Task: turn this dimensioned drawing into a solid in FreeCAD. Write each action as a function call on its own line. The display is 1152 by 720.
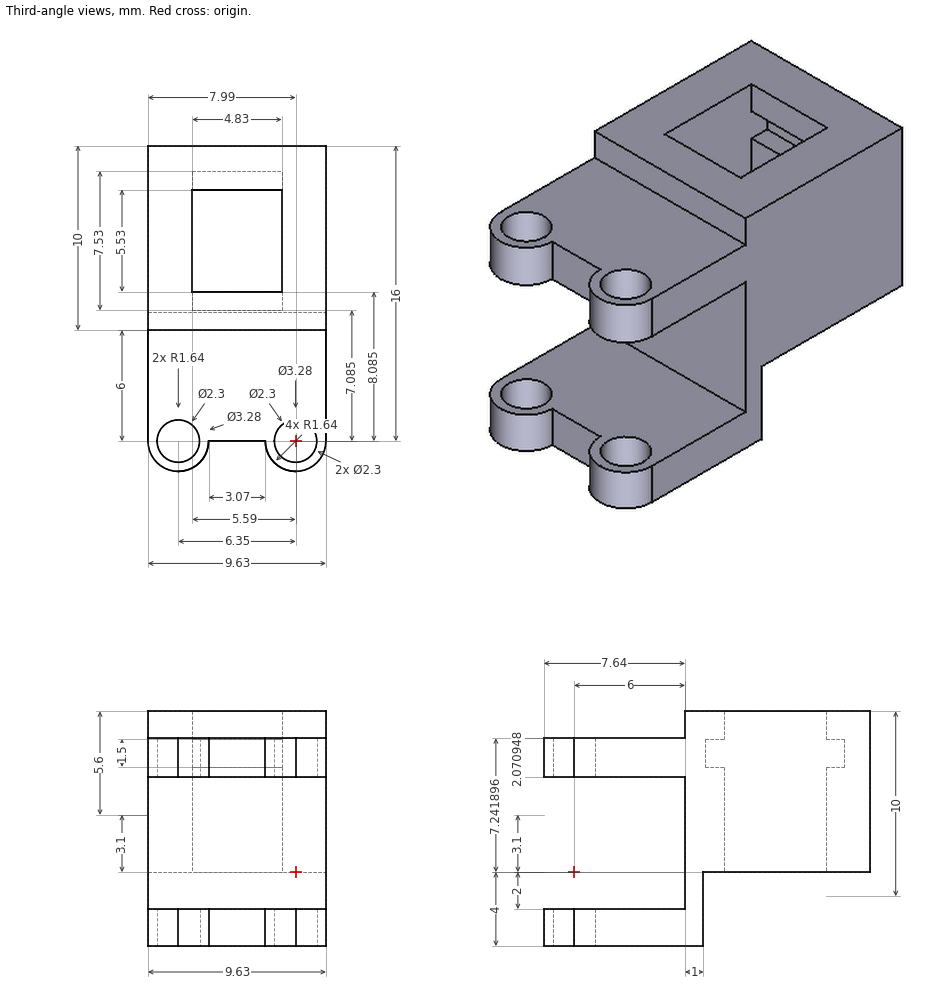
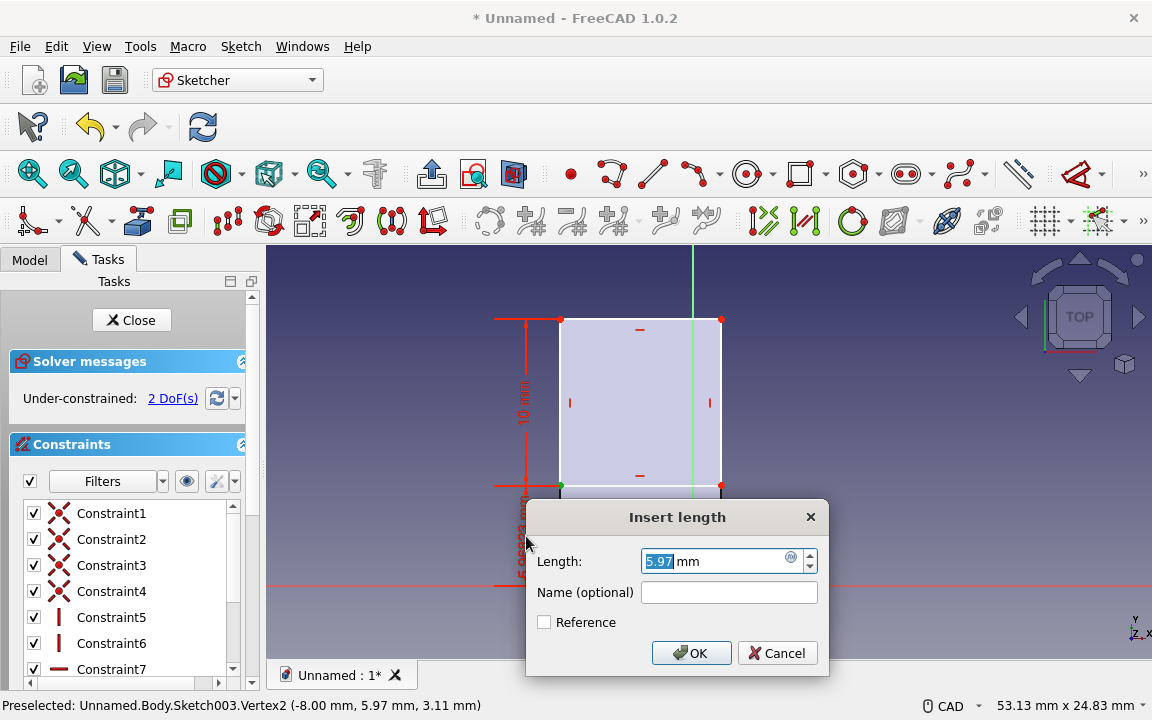
text(6)
key(Return)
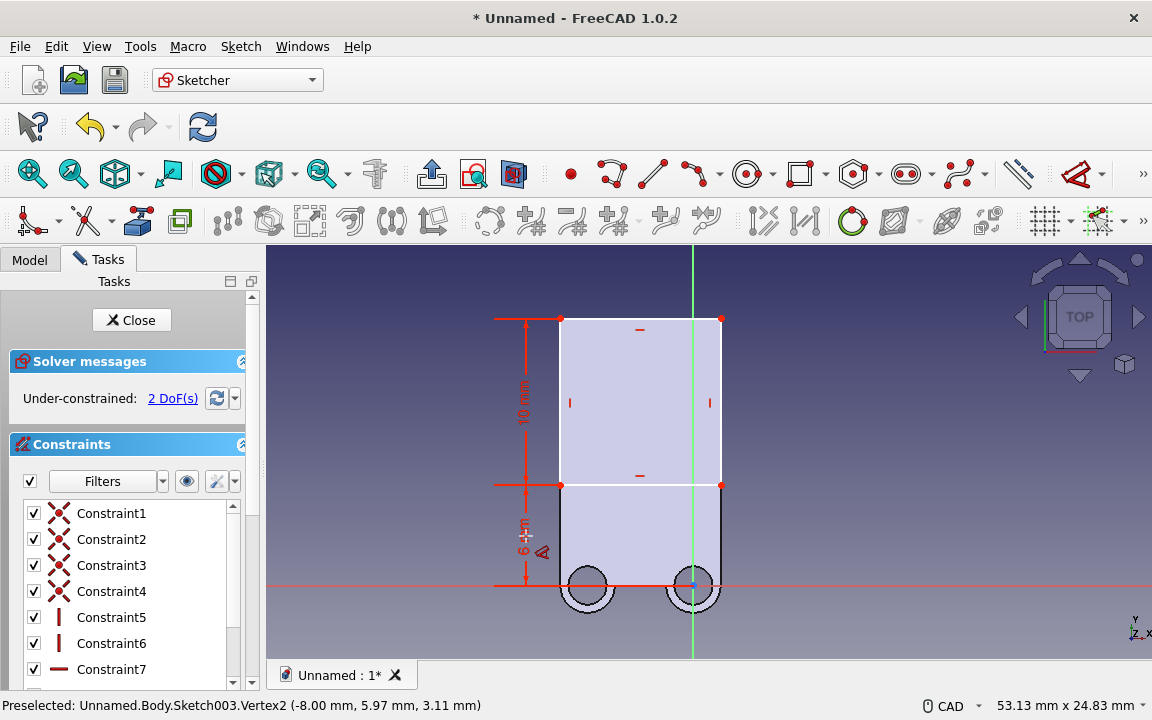
click(608, 485)
click(640, 519)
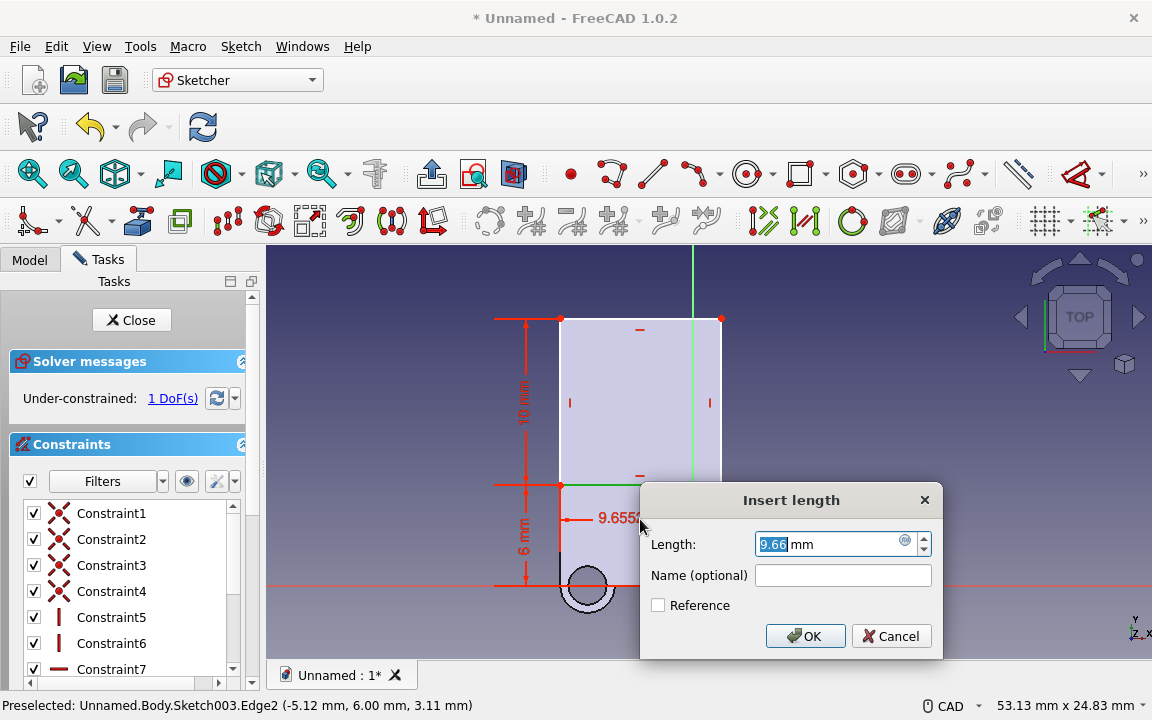
text(9.63)
key(Return)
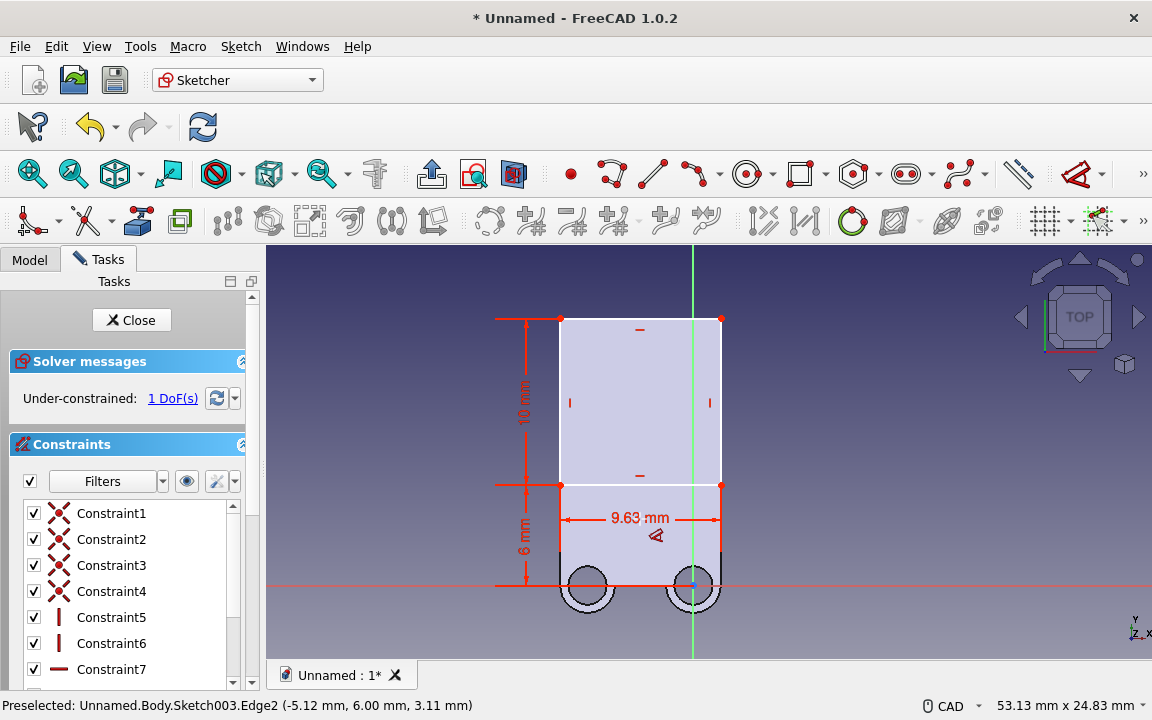
click(560, 319)
click(627, 620)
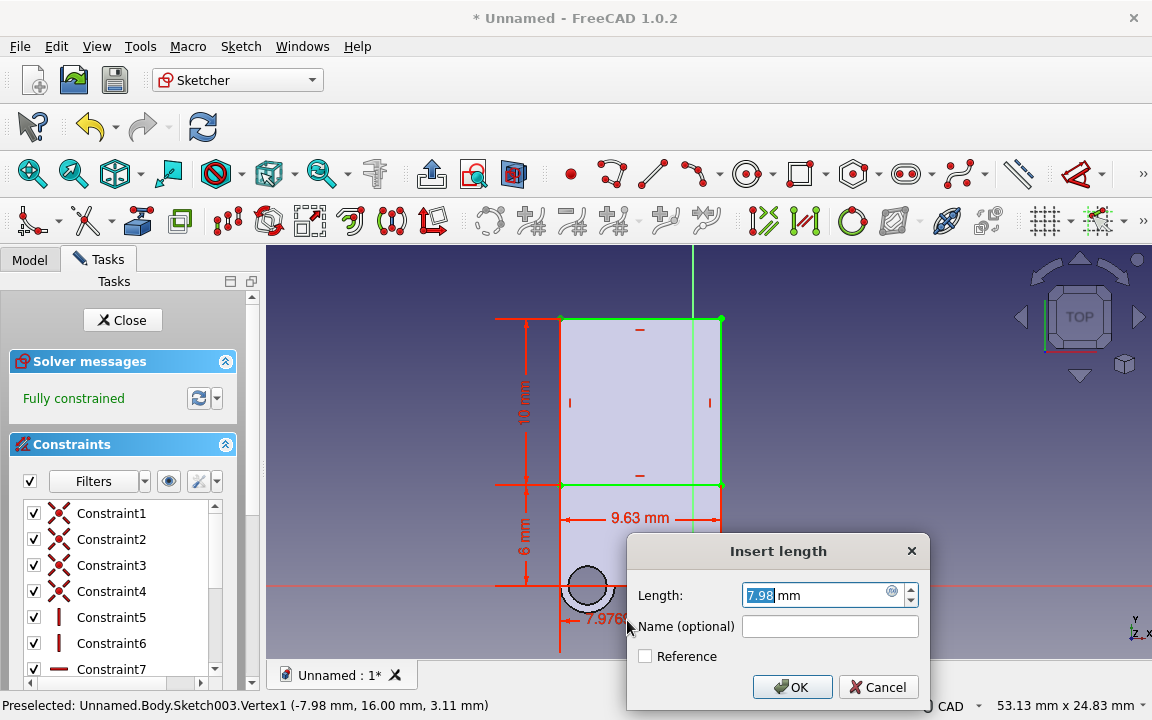
text(7.99)
key(Return)
key(Escape)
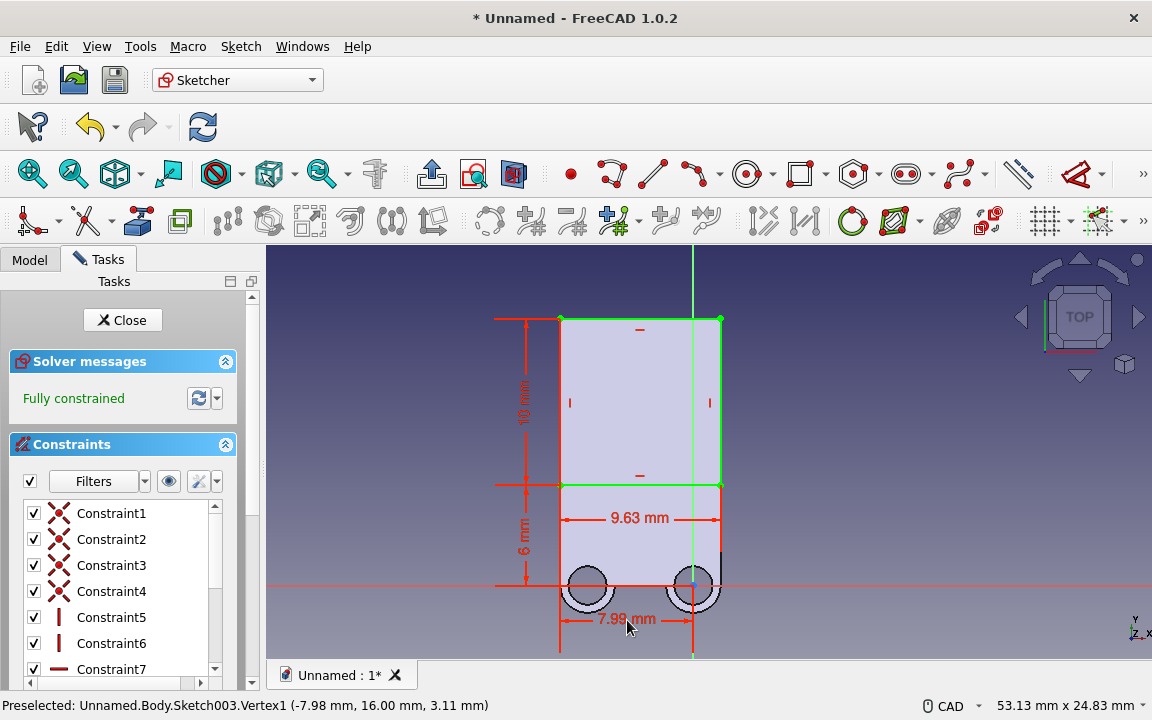
click(123, 320)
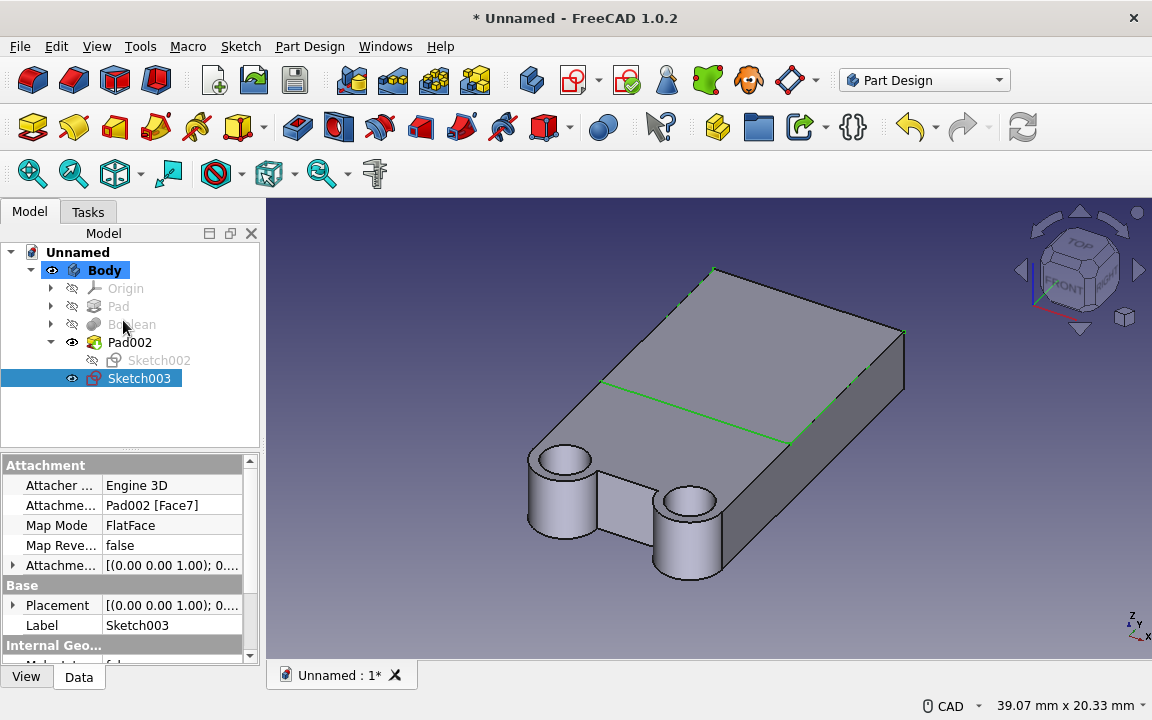
click(33, 128)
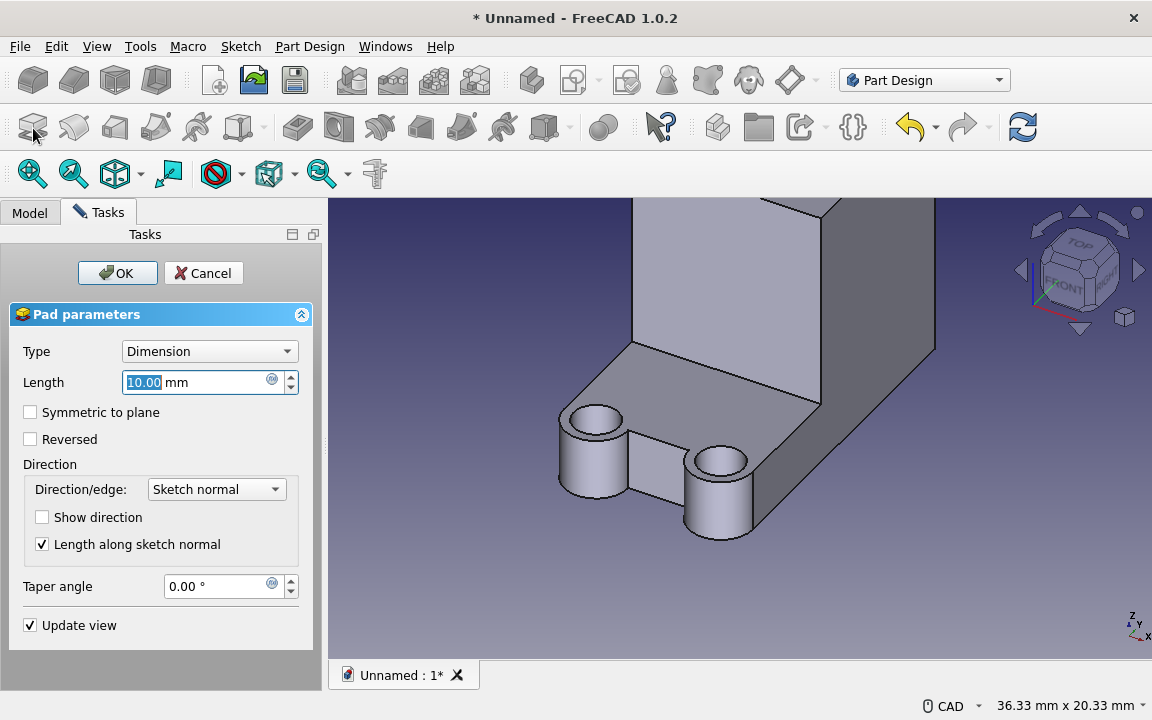
text(5.6)
key(Tab)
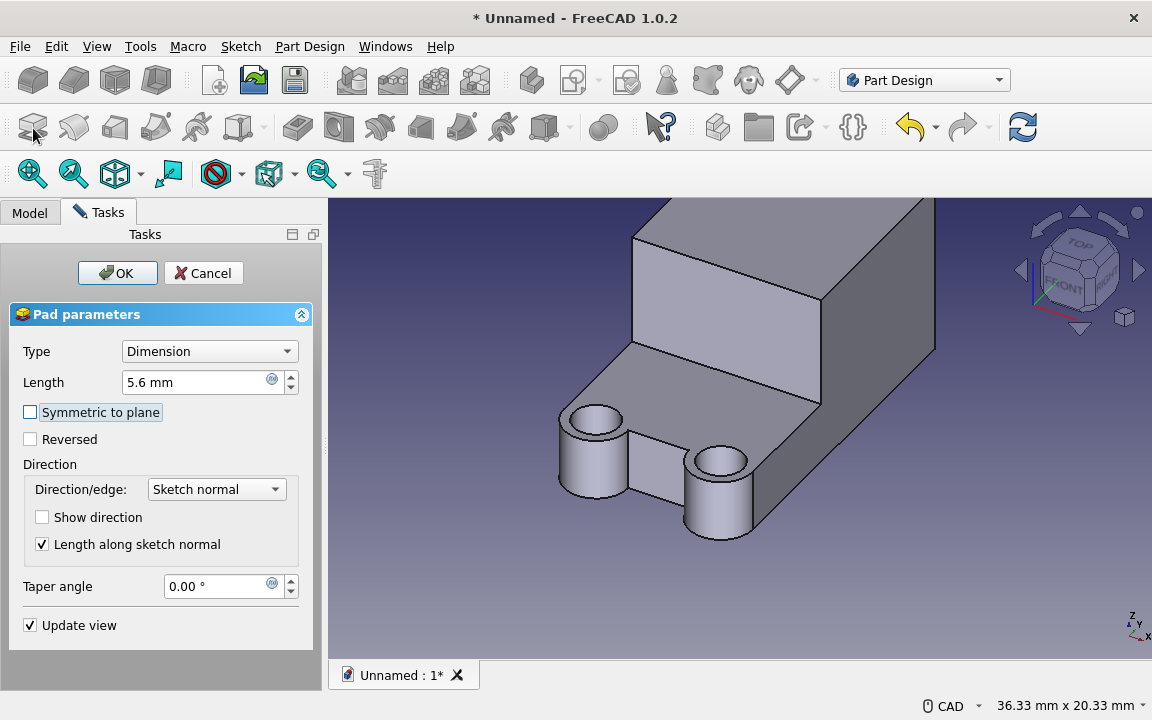
click(118, 273)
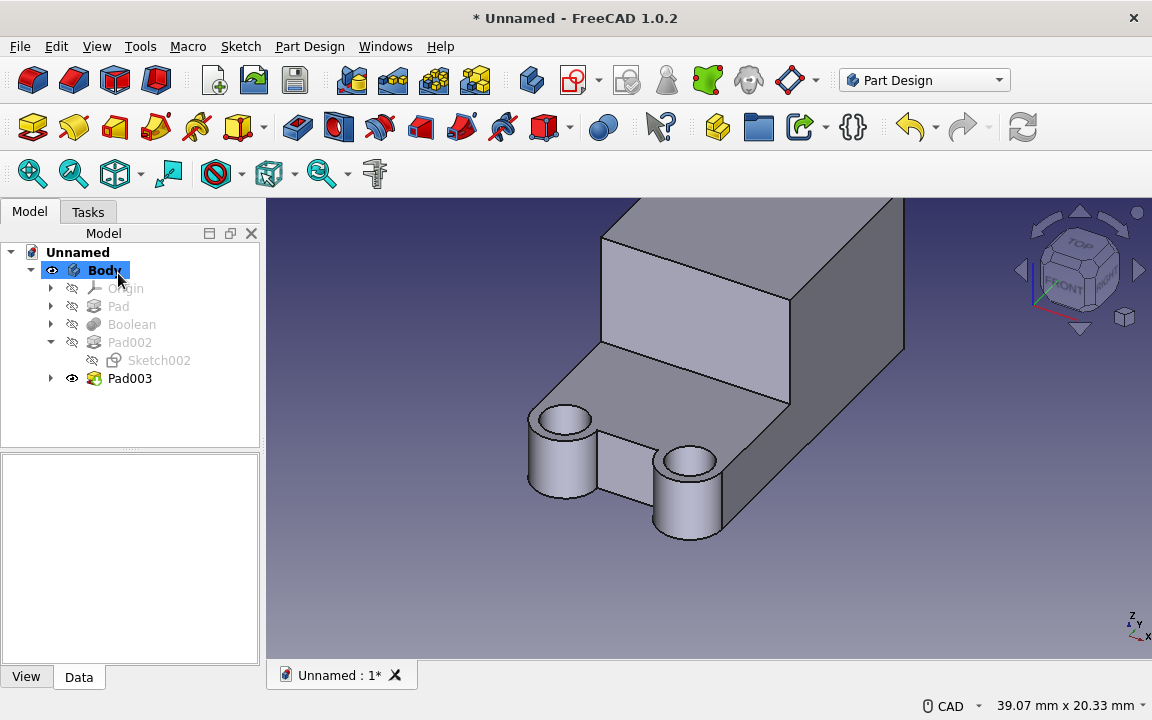
key(v)
key(f)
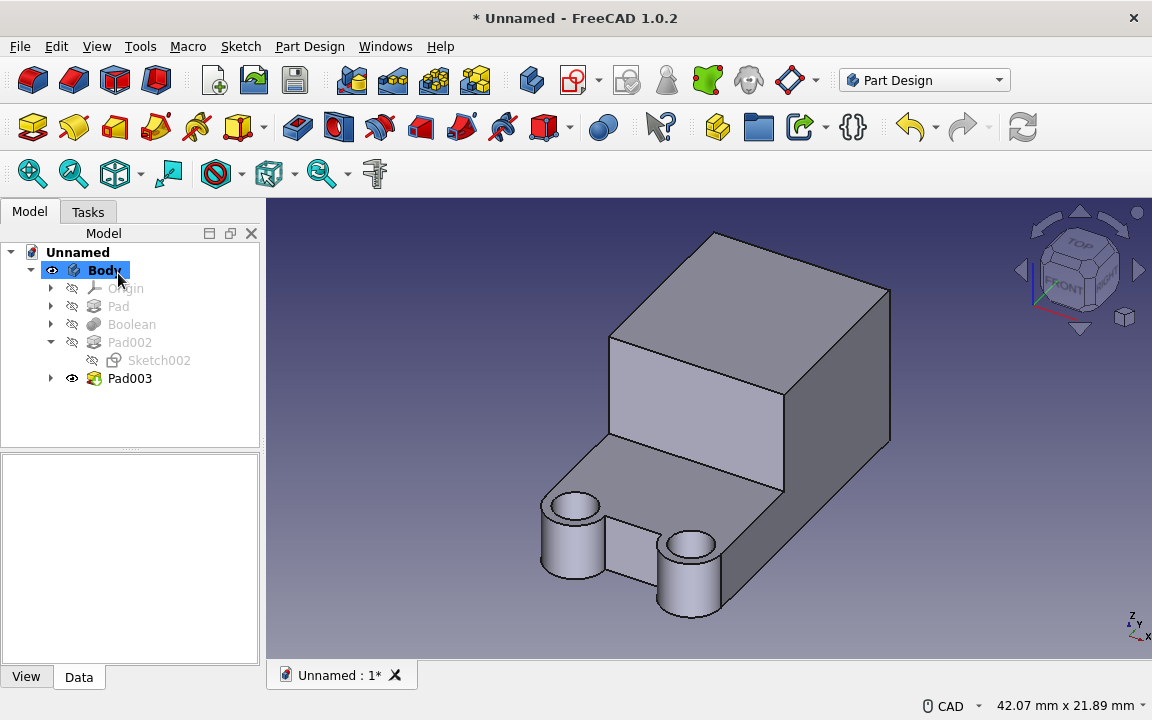
click(749, 313)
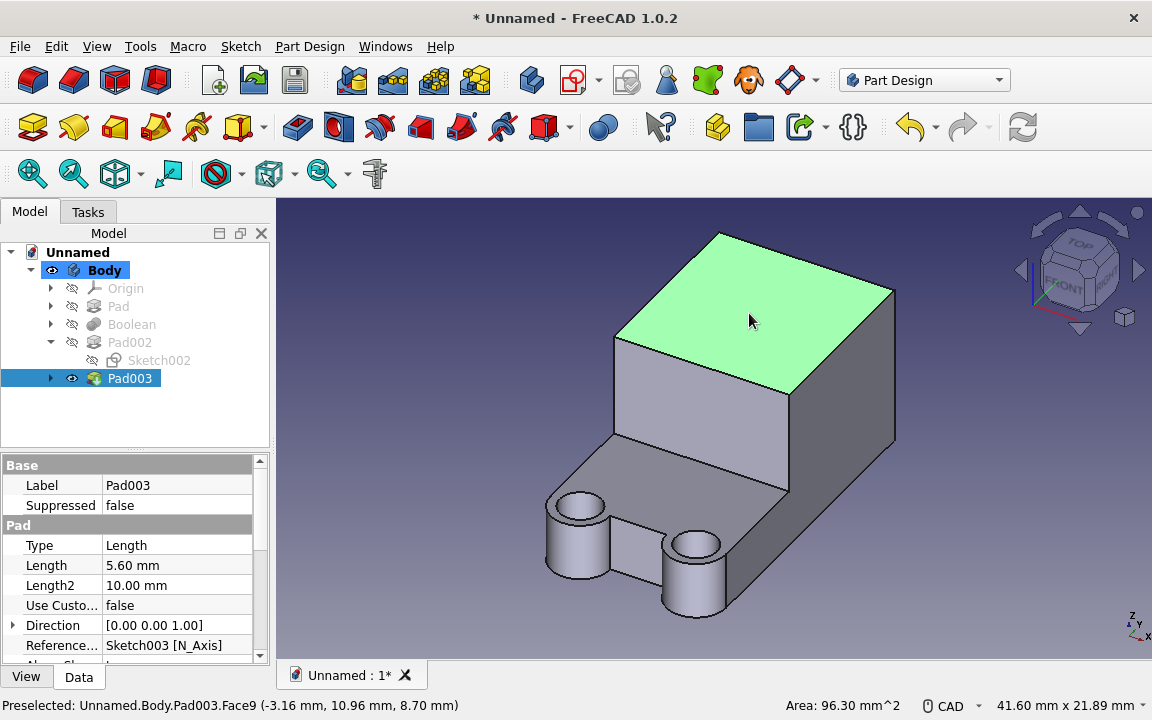
click(572, 80)